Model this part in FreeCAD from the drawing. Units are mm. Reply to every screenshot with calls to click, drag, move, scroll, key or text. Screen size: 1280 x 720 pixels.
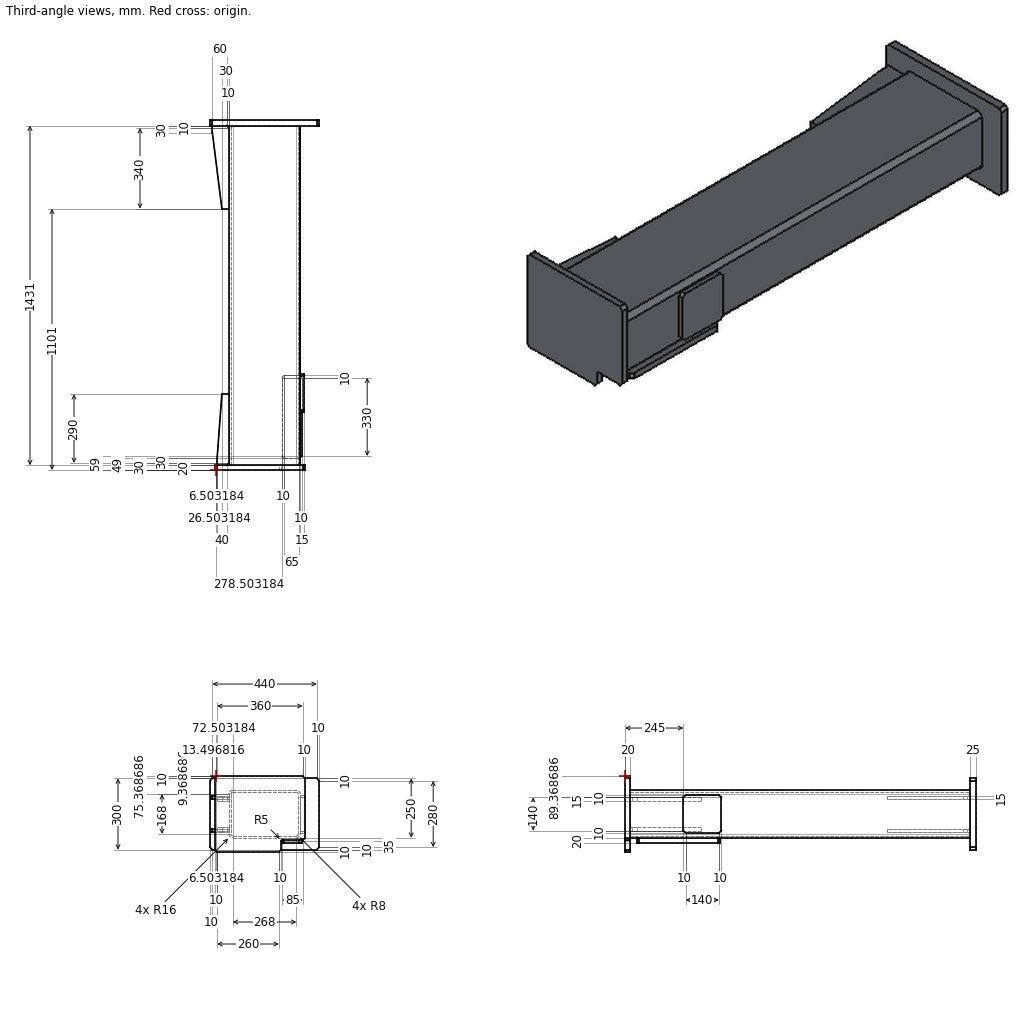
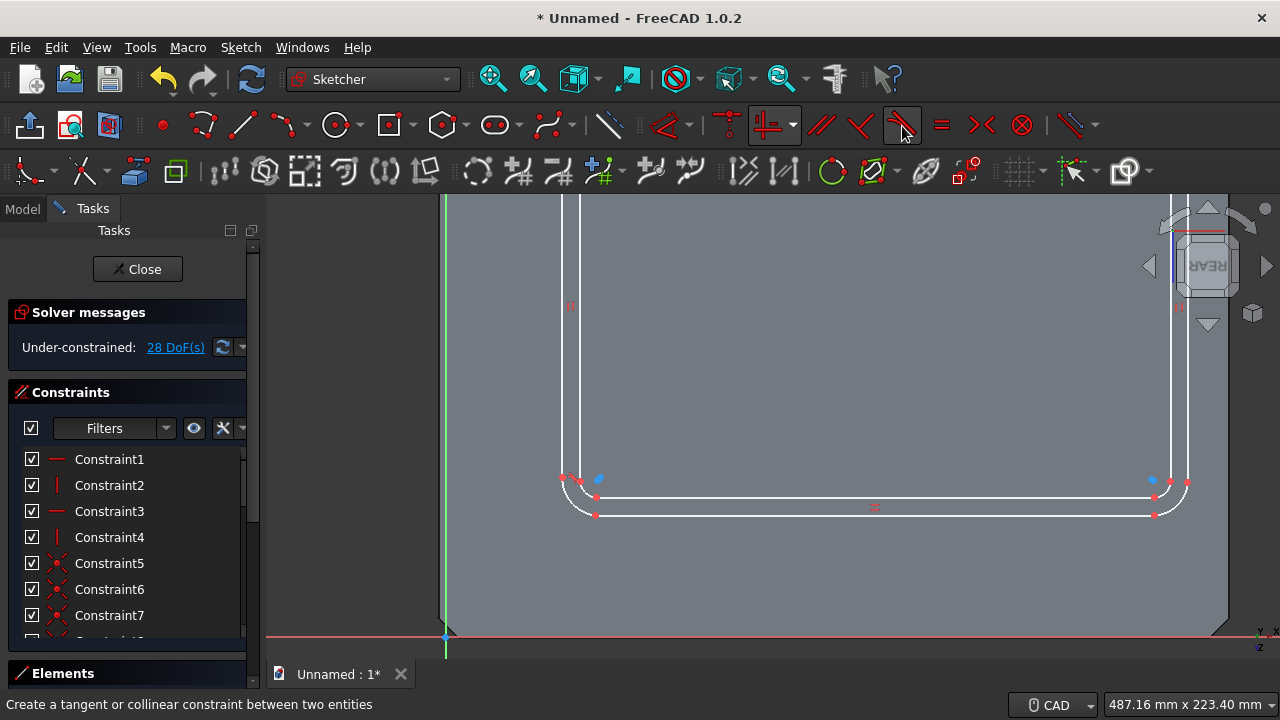
click(763, 516)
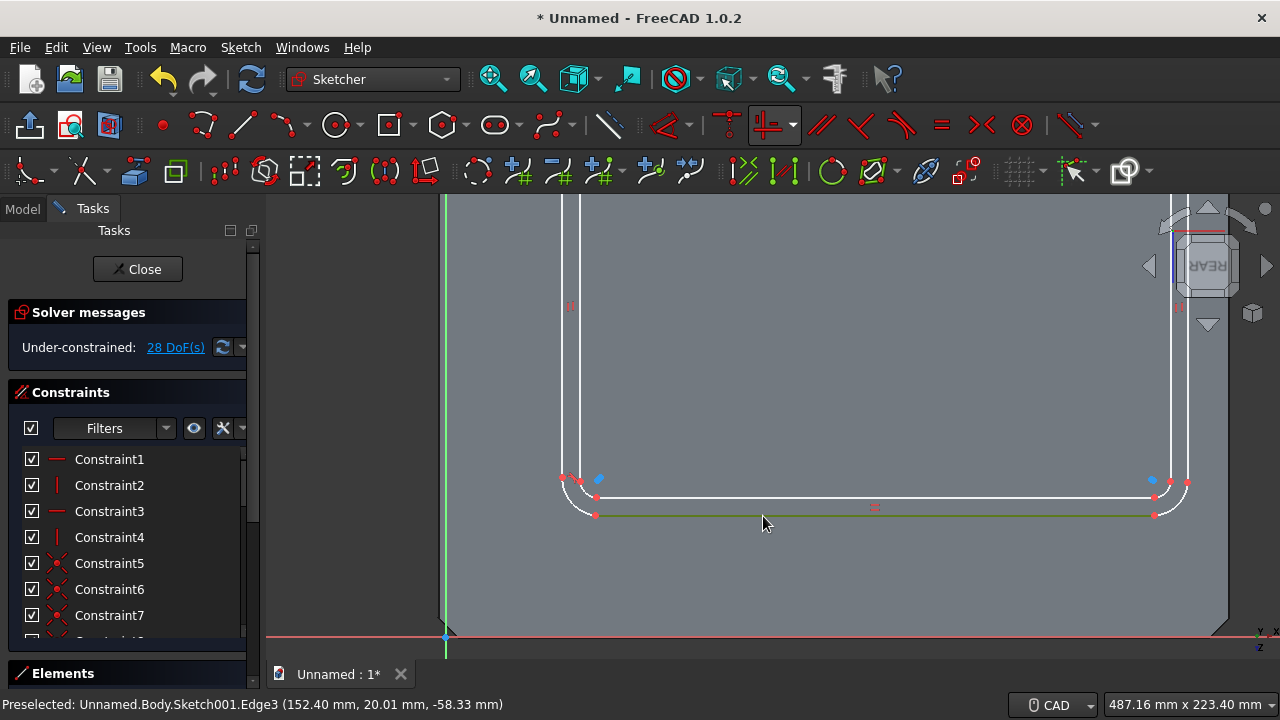
click(566, 494)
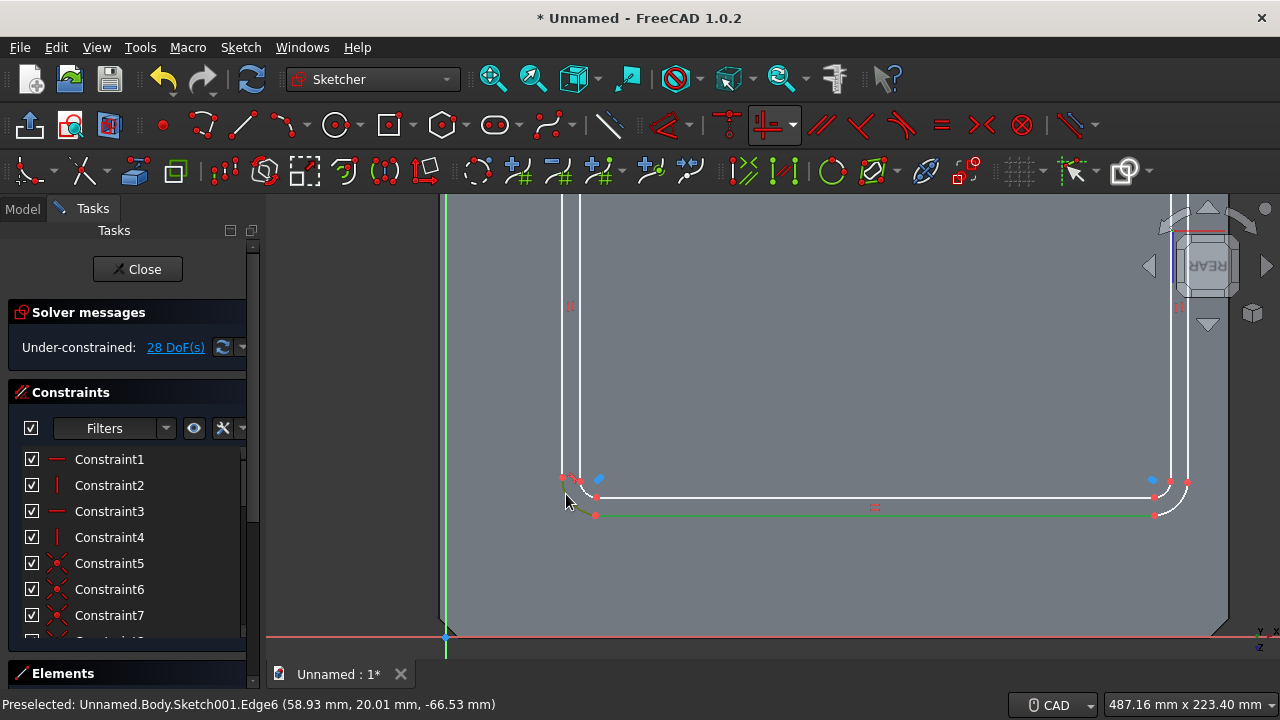
click(902, 126)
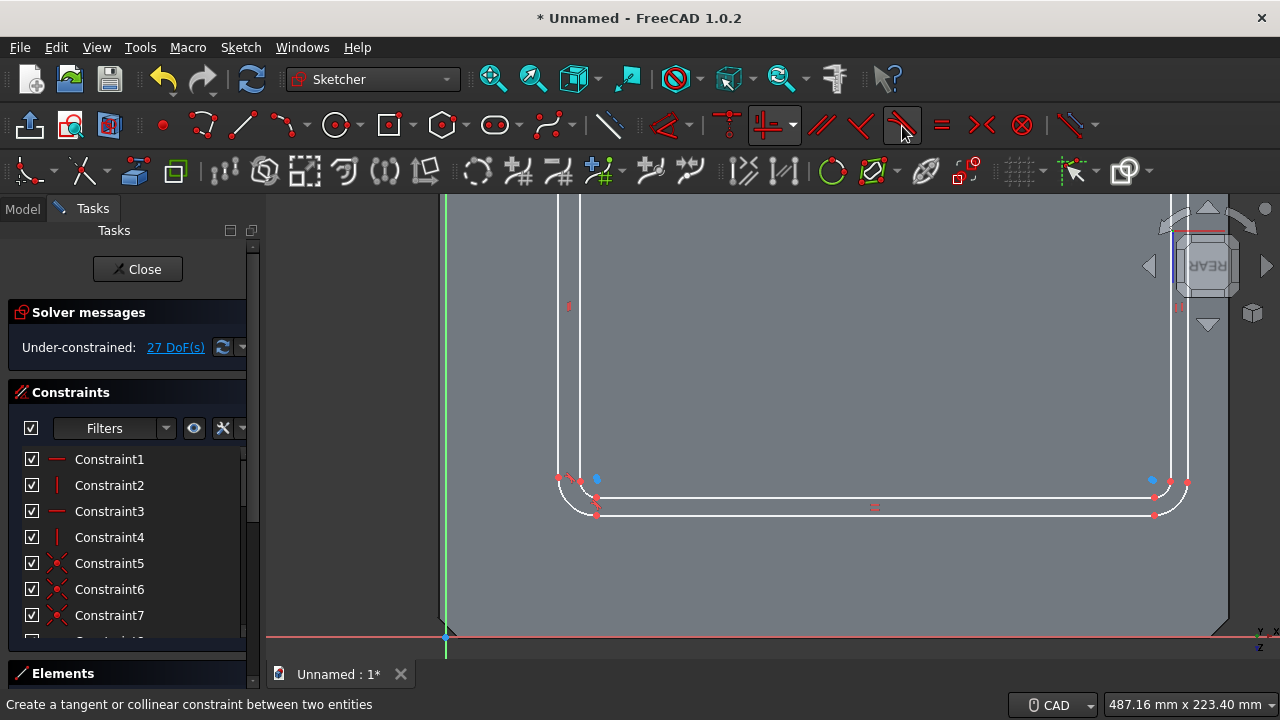
click(764, 516)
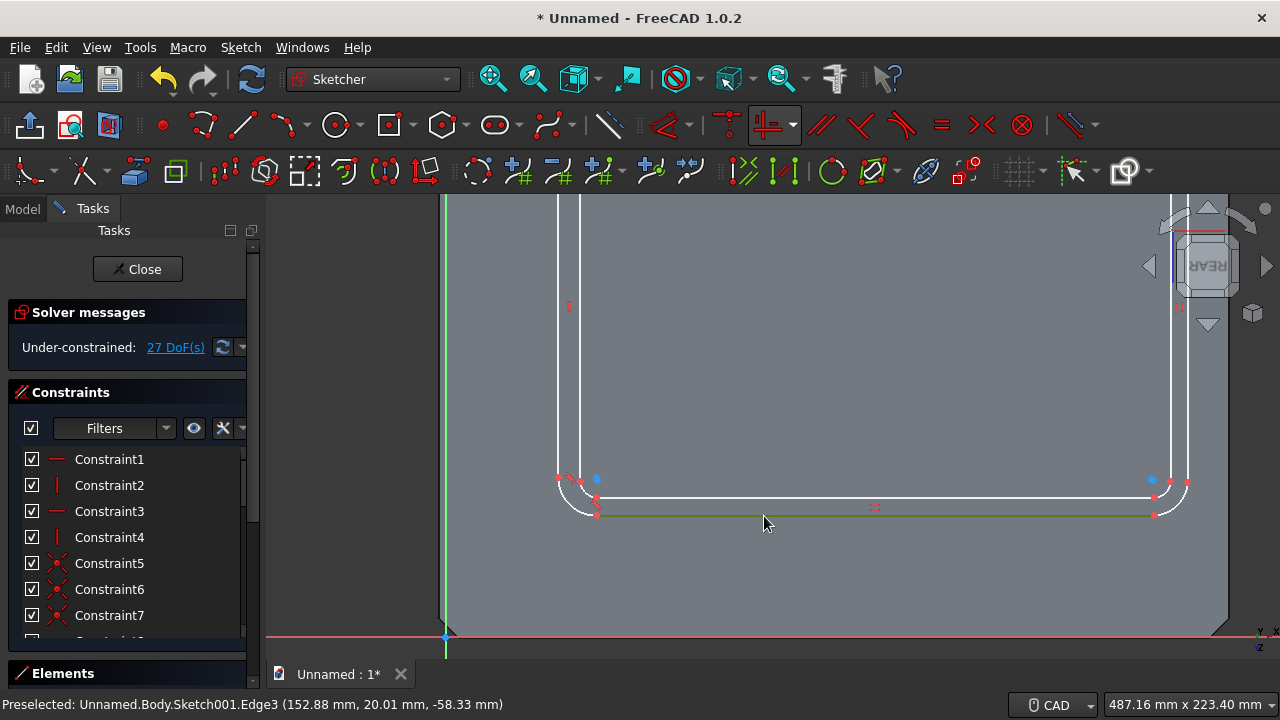
scroll(568, 499, down, 3)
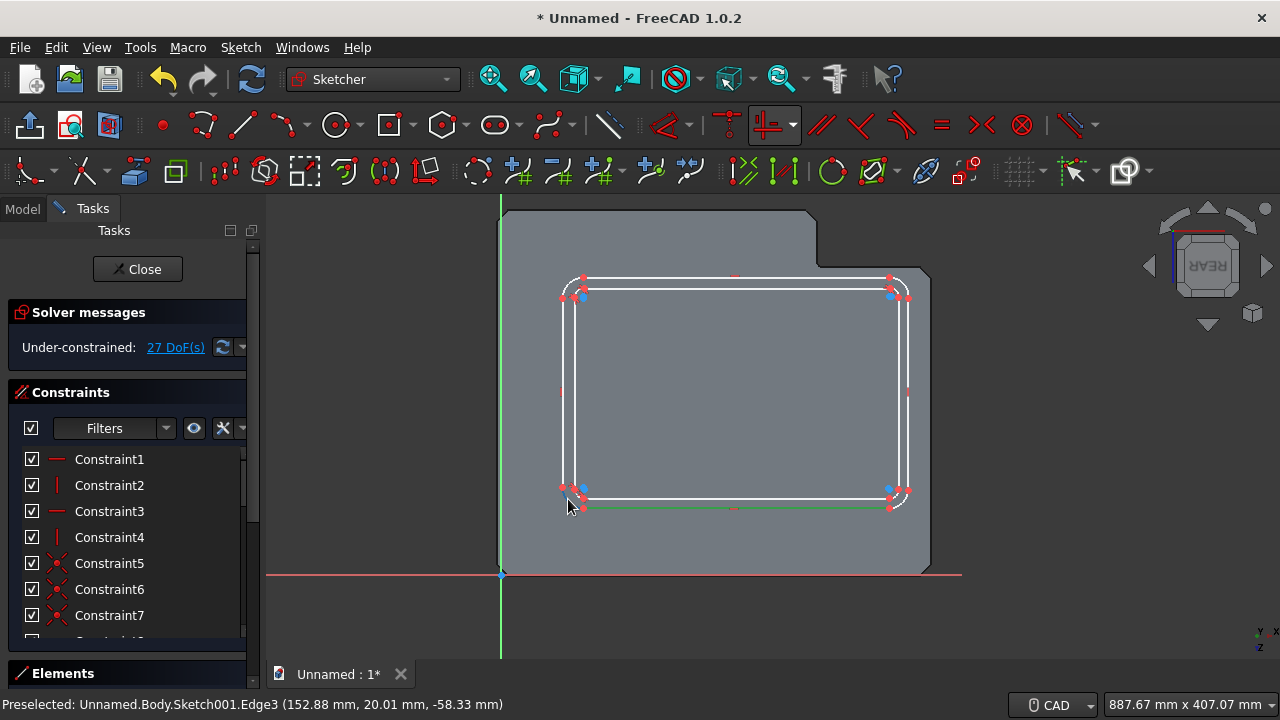
scroll(898, 506, up, 3)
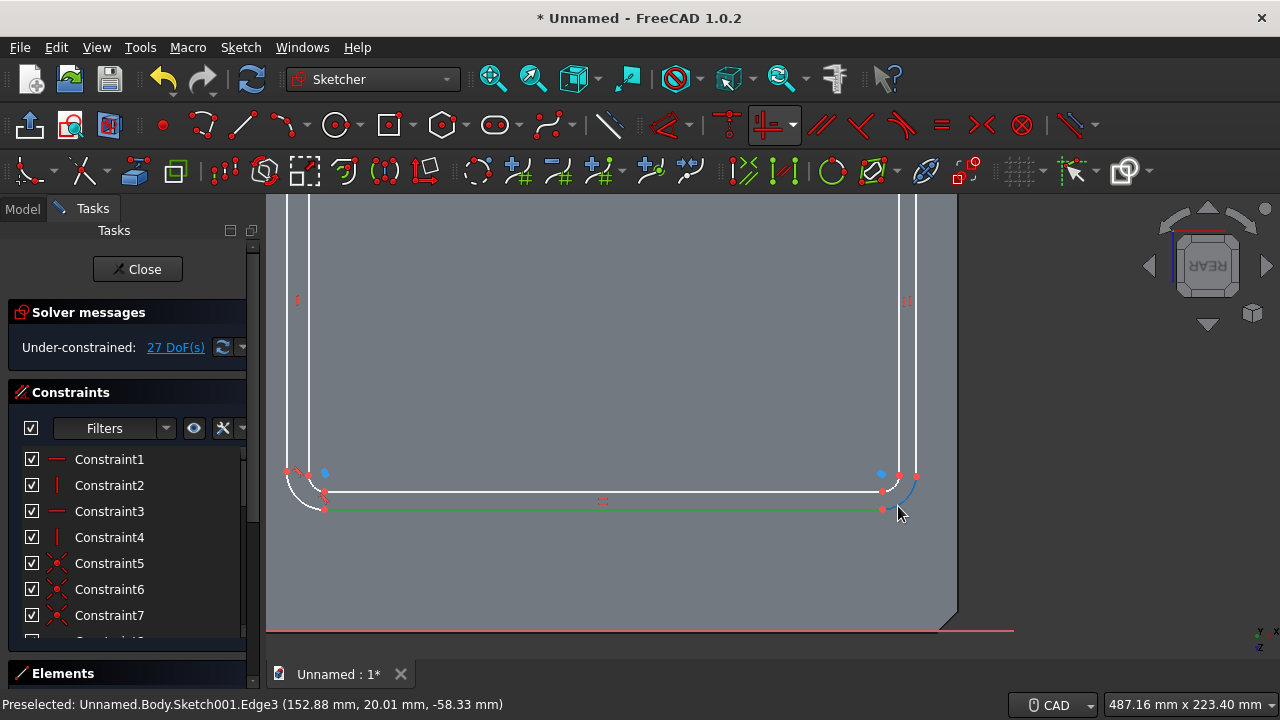
click(898, 506)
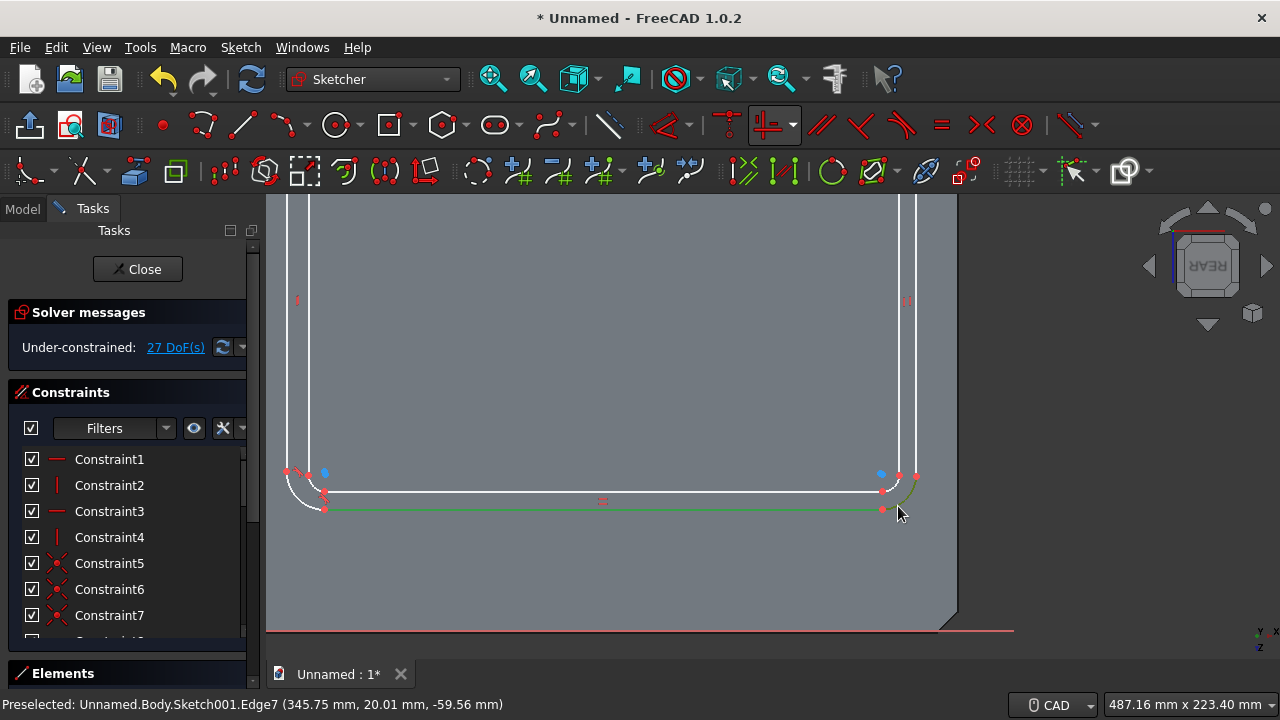
key(t)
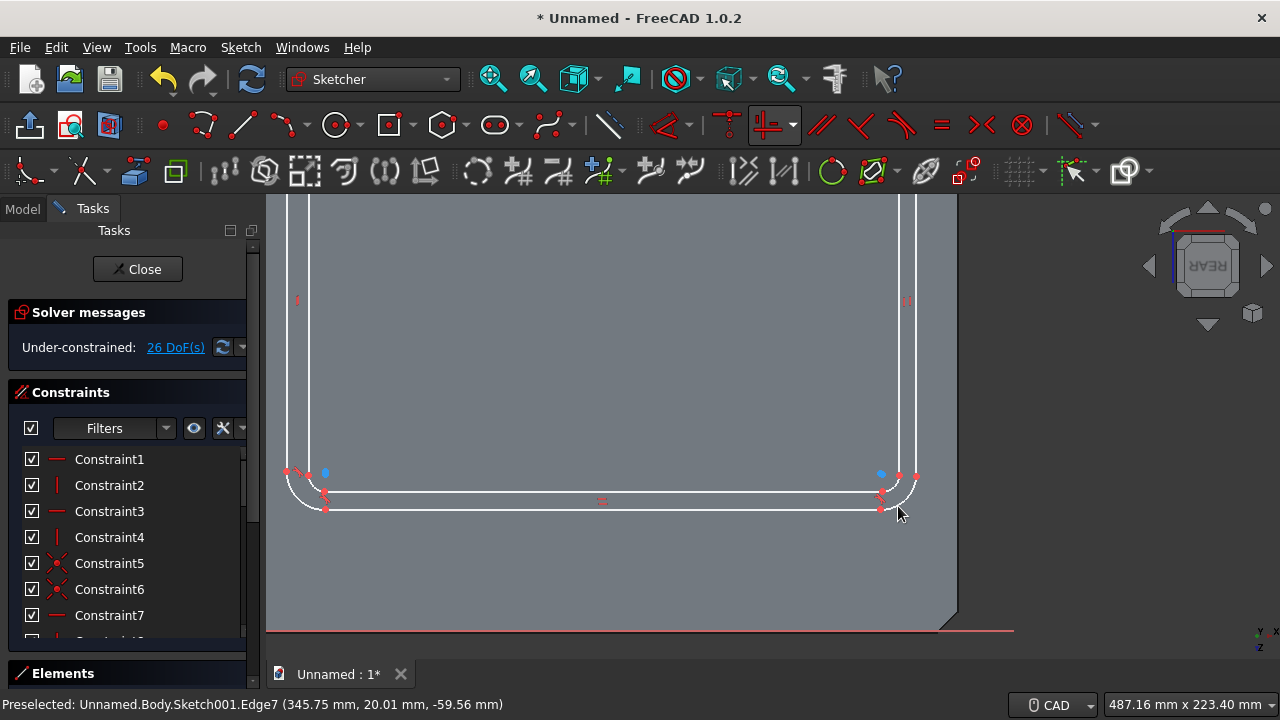
click(916, 372)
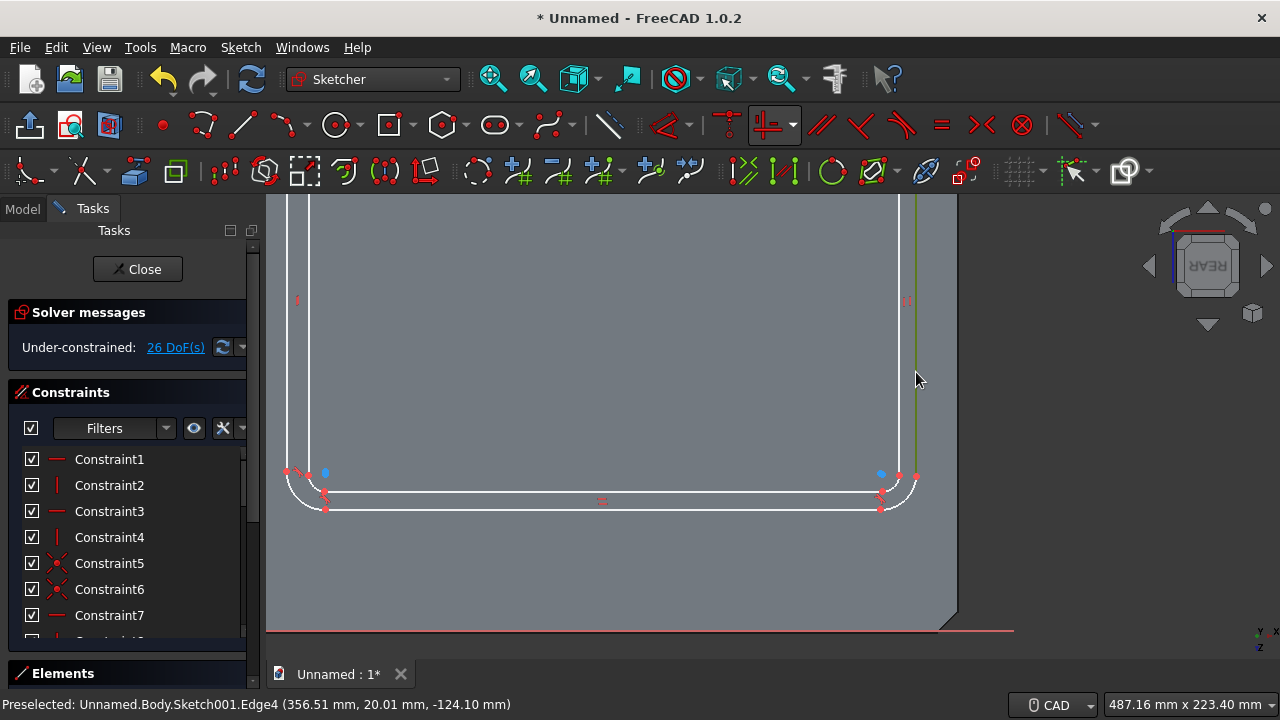
click(896, 506)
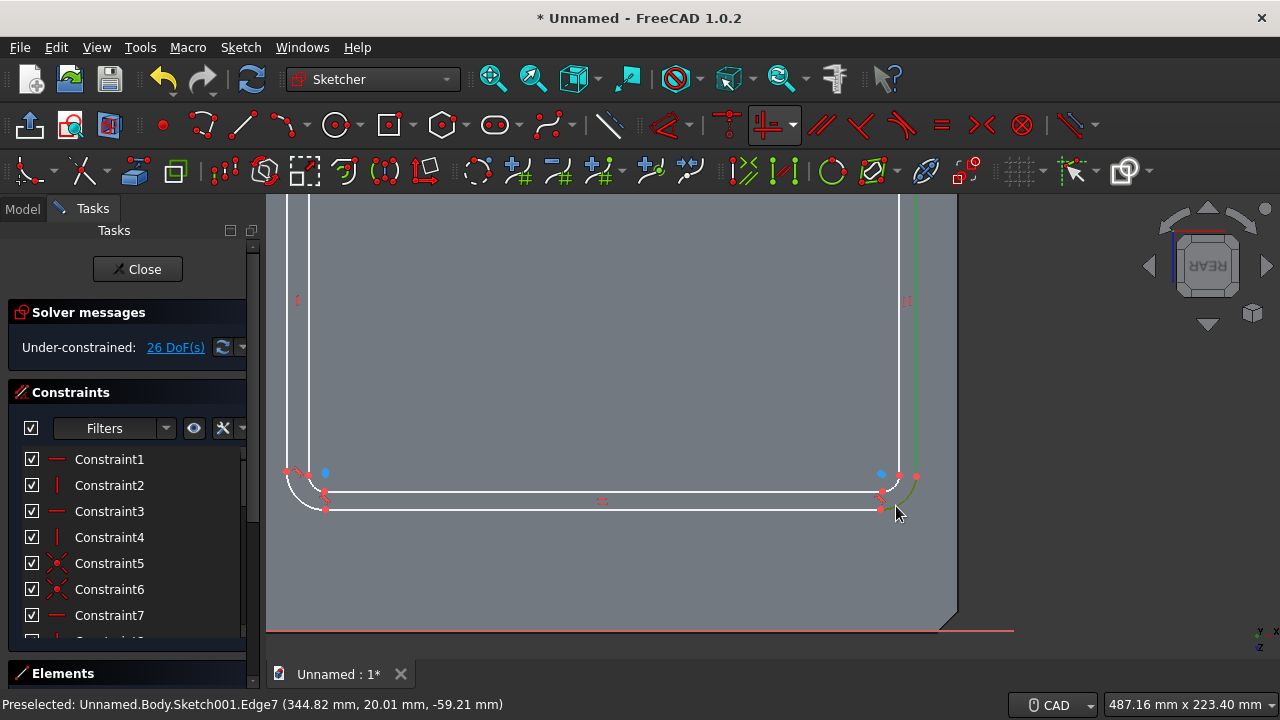
click(902, 126)